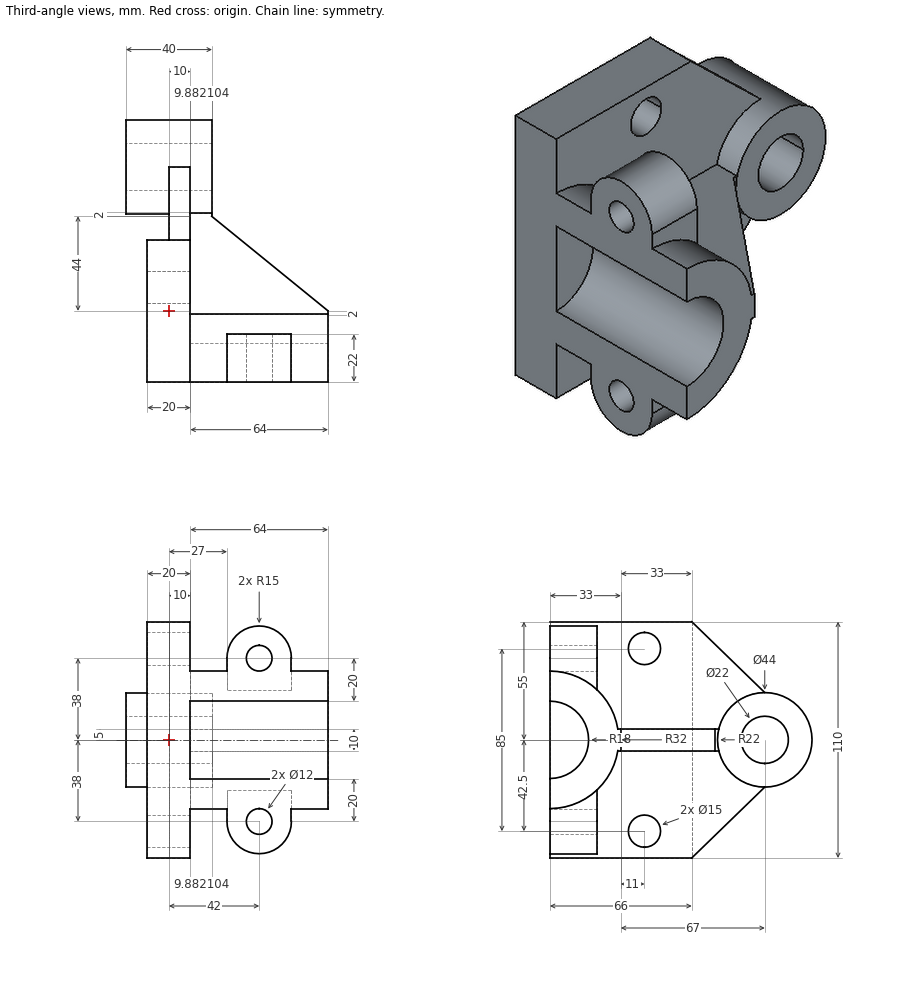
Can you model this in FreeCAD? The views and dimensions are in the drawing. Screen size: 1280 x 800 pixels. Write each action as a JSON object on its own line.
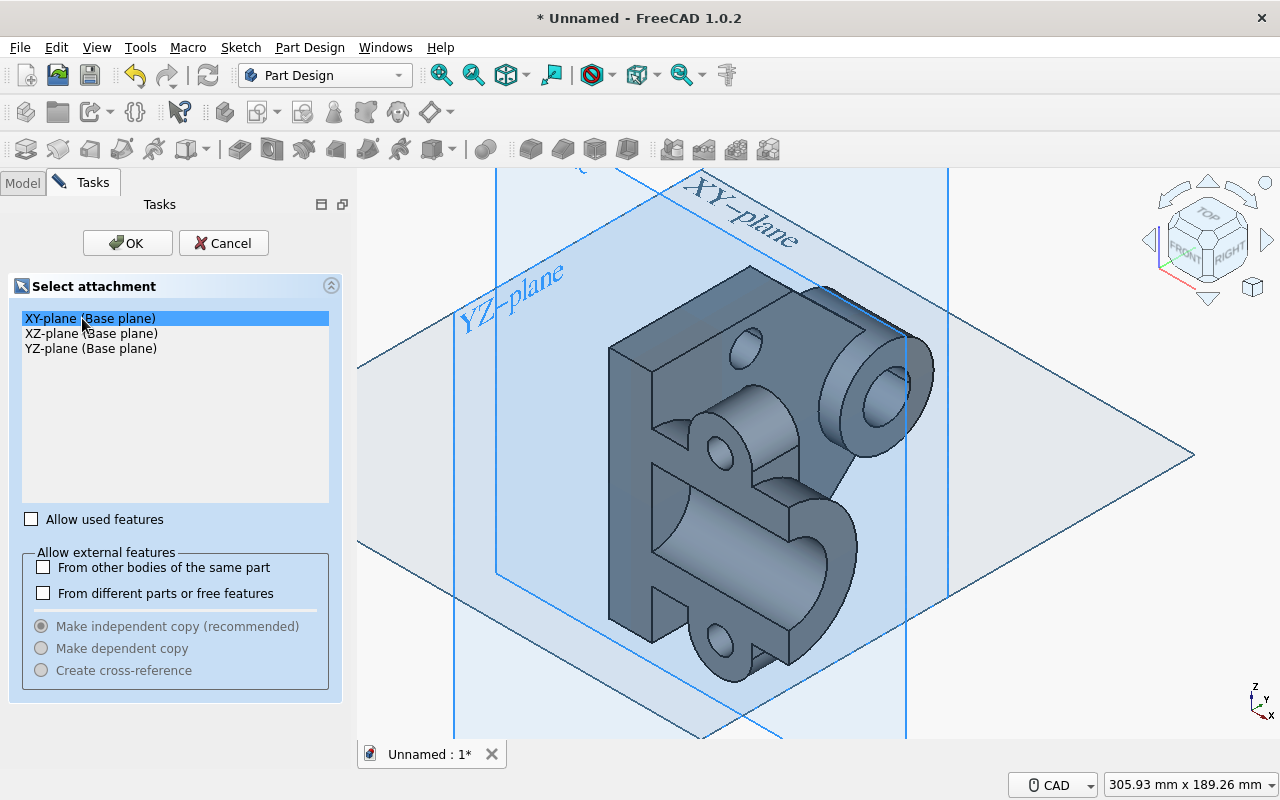
{"action": "left_click", "coordinate": [128, 243]}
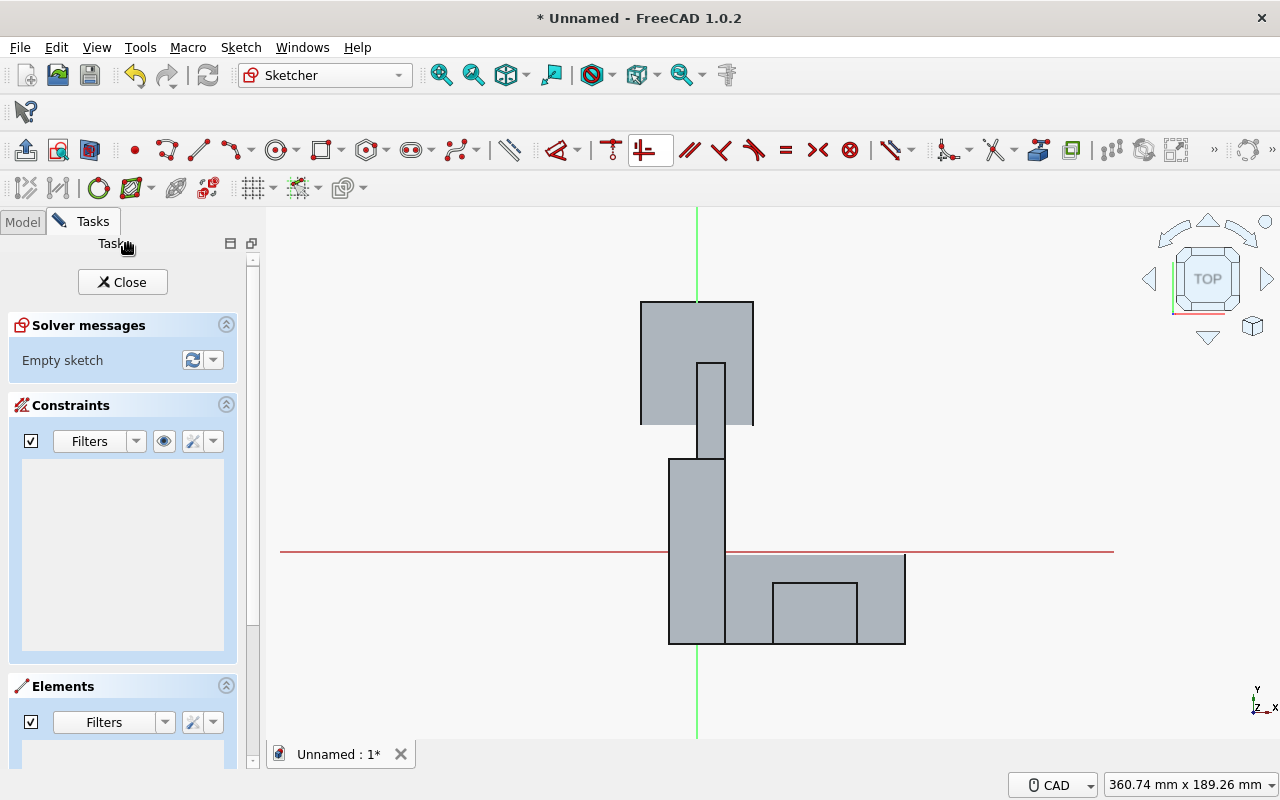
{"action": "left_click", "coordinate": [90, 150]}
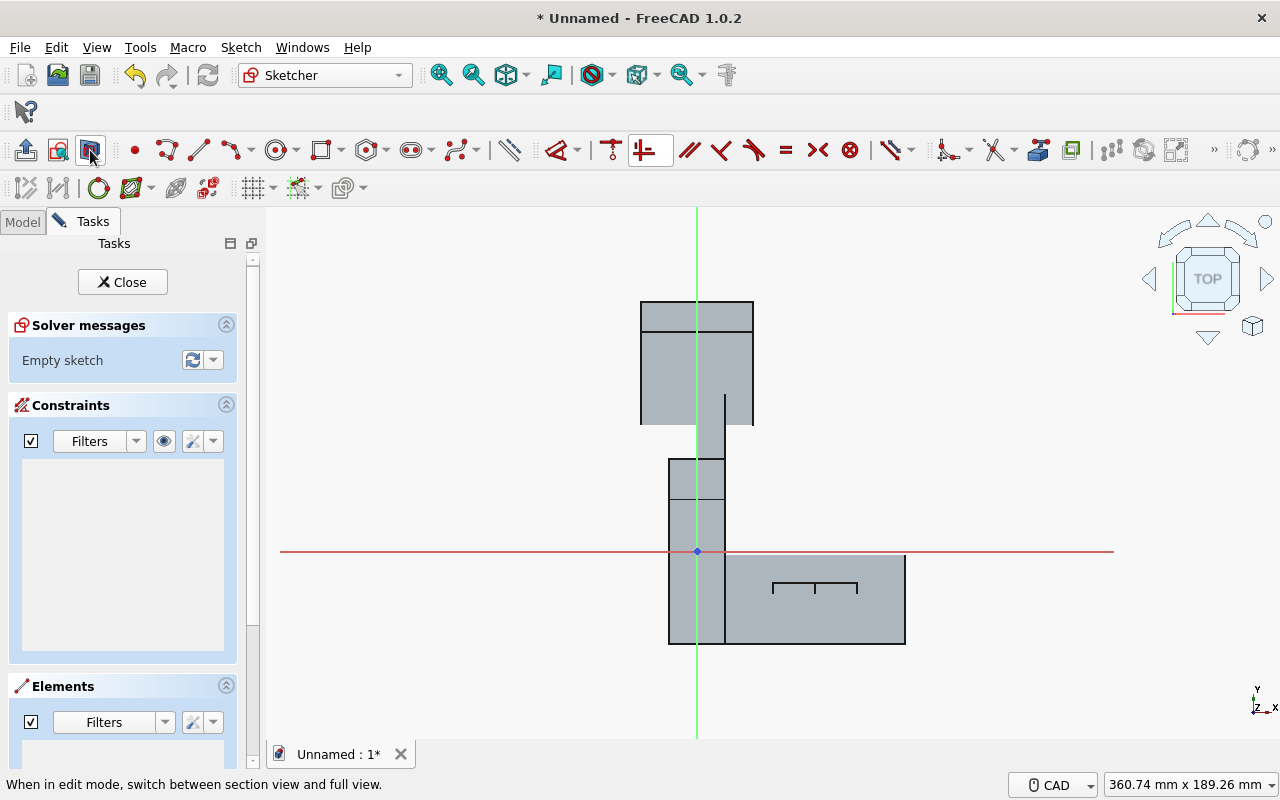
{"action": "scroll", "coordinate": [857, 500], "scroll_direction": "up", "scroll_amount": 5}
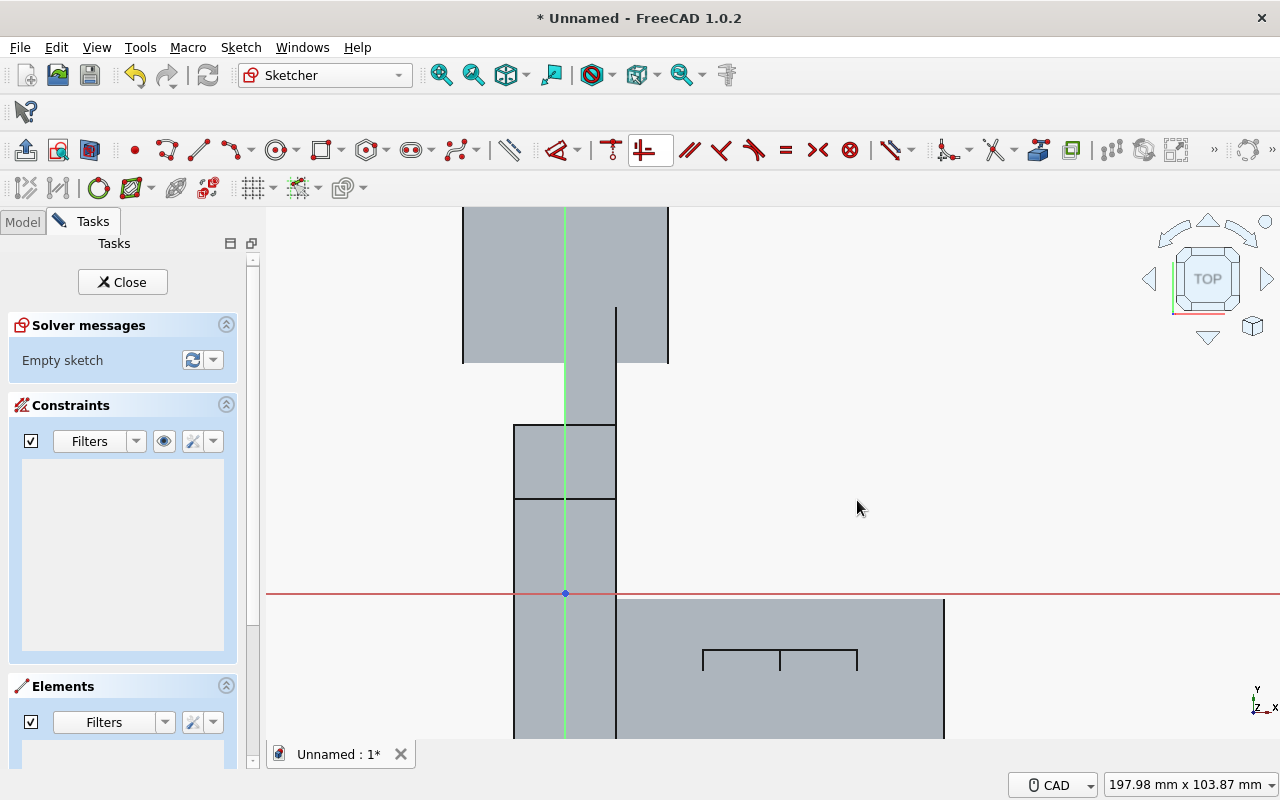
{"action": "left_click", "coordinate": [168, 150]}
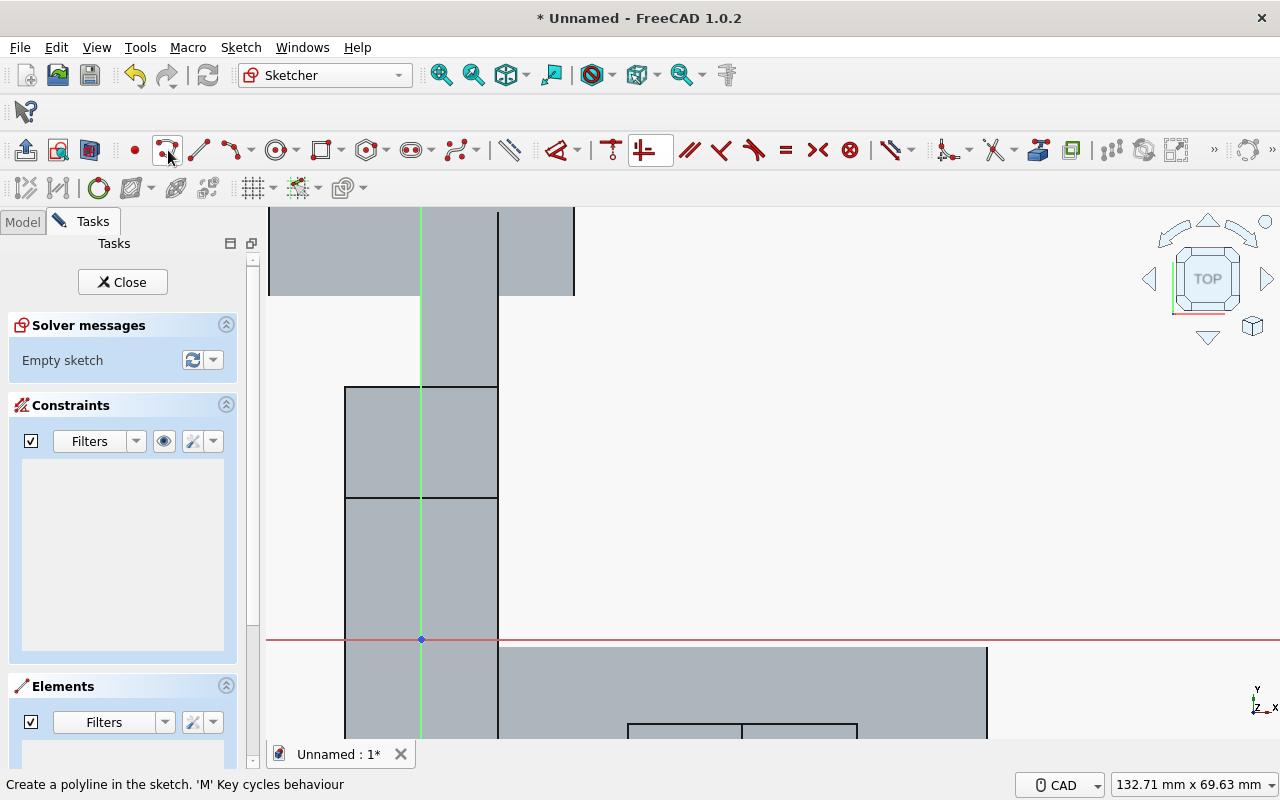
{"action": "left_click", "coordinate": [498, 640]}
{"action": "left_click", "coordinate": [987, 631]}
{"action": "left_click", "coordinate": [573, 303]}
{"action": "left_click", "coordinate": [498, 303]}
{"action": "left_click", "coordinate": [498, 640]}
{"action": "key", "text": "Escape"}
{"action": "key", "text": "Escape"}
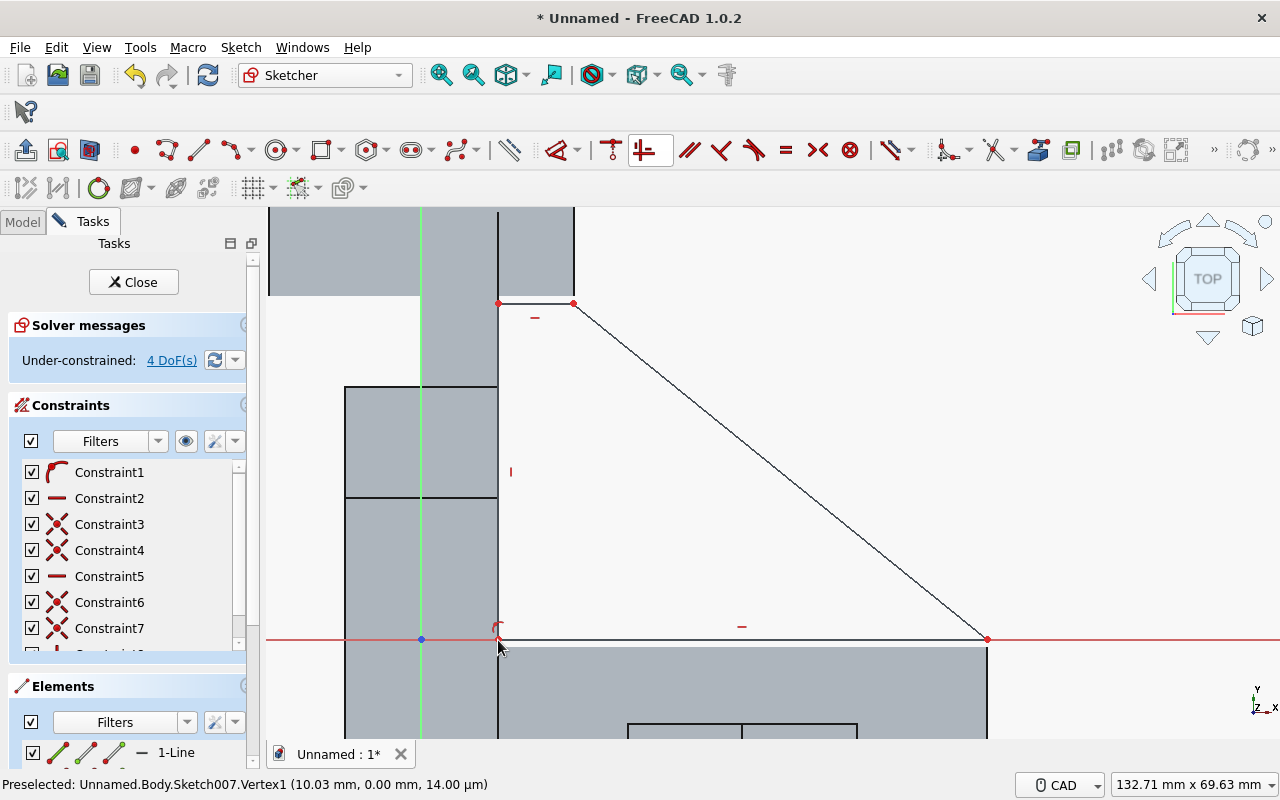
{"action": "left_click", "coordinate": [556, 150]}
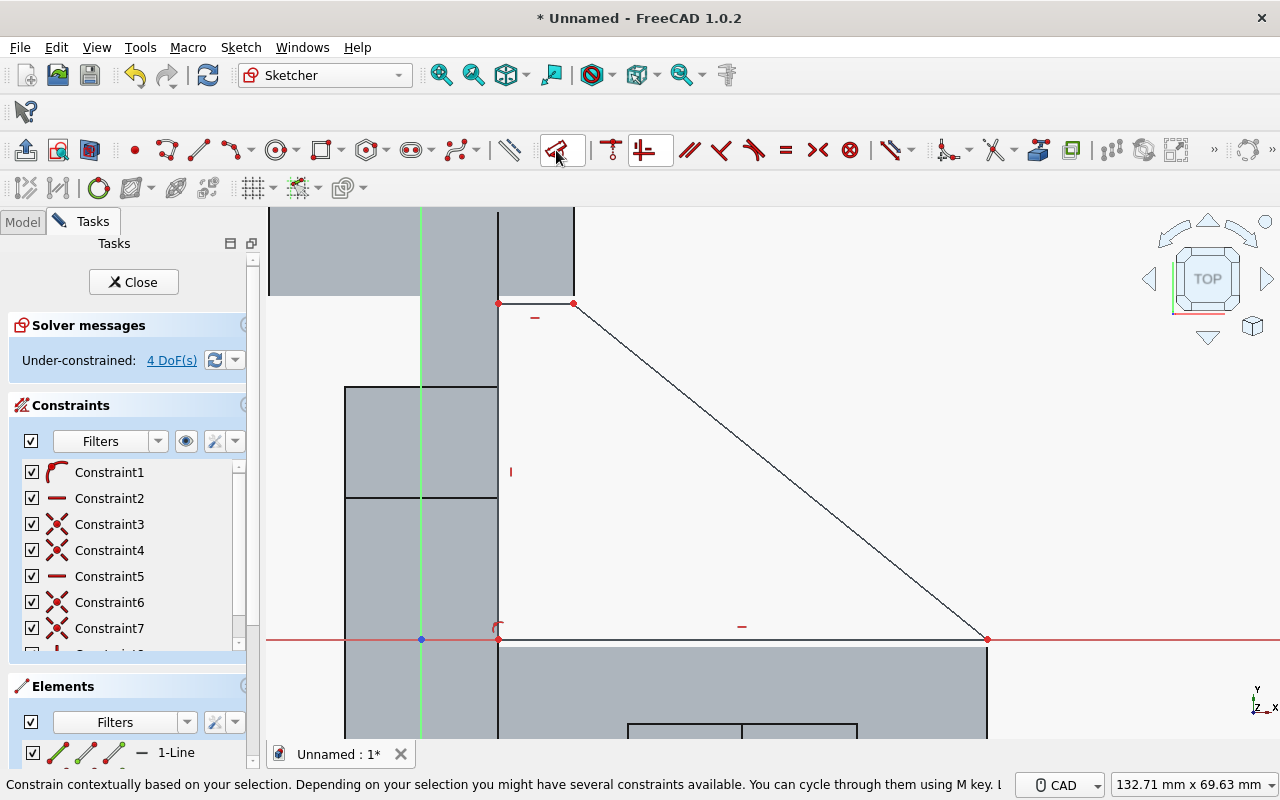
{"action": "left_click", "coordinate": [645, 640]}
{"action": "left_click", "coordinate": [743, 674]}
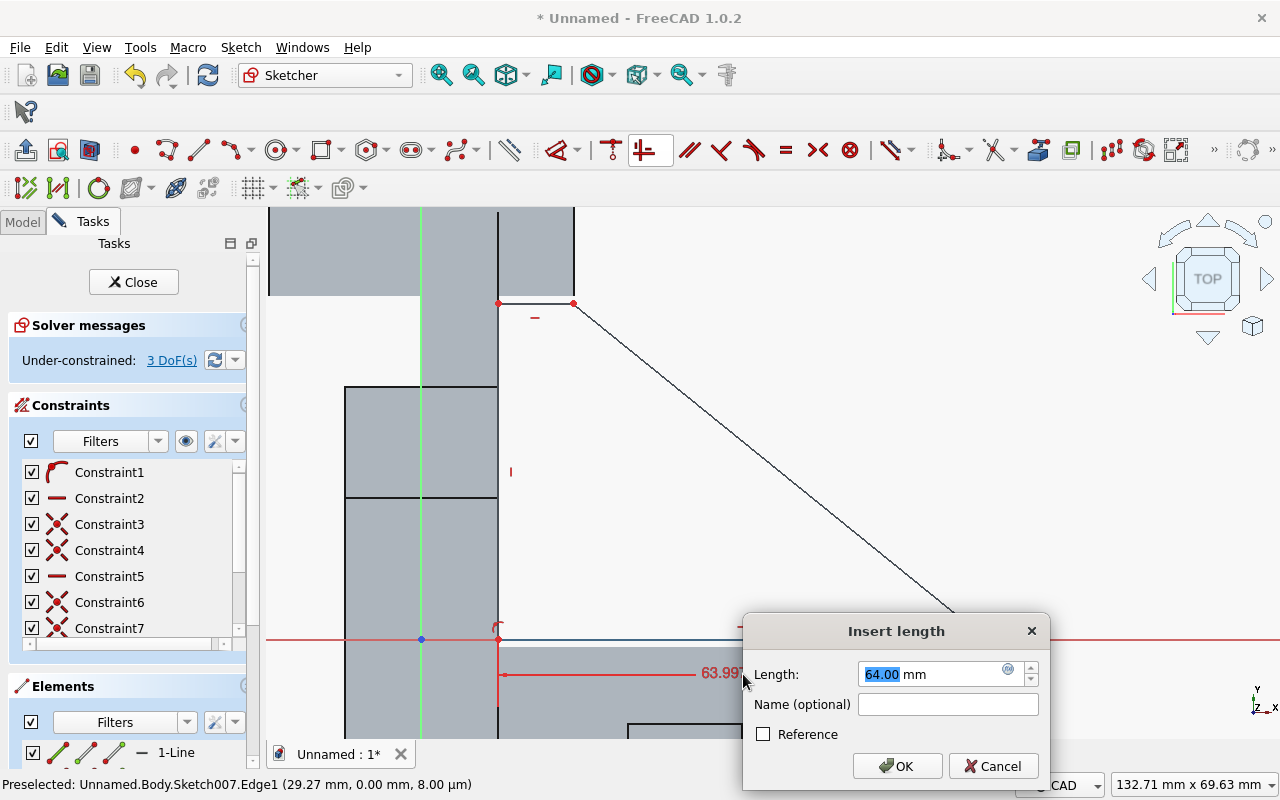
{"action": "type", "text": "64"}
{"action": "key", "text": "Return"}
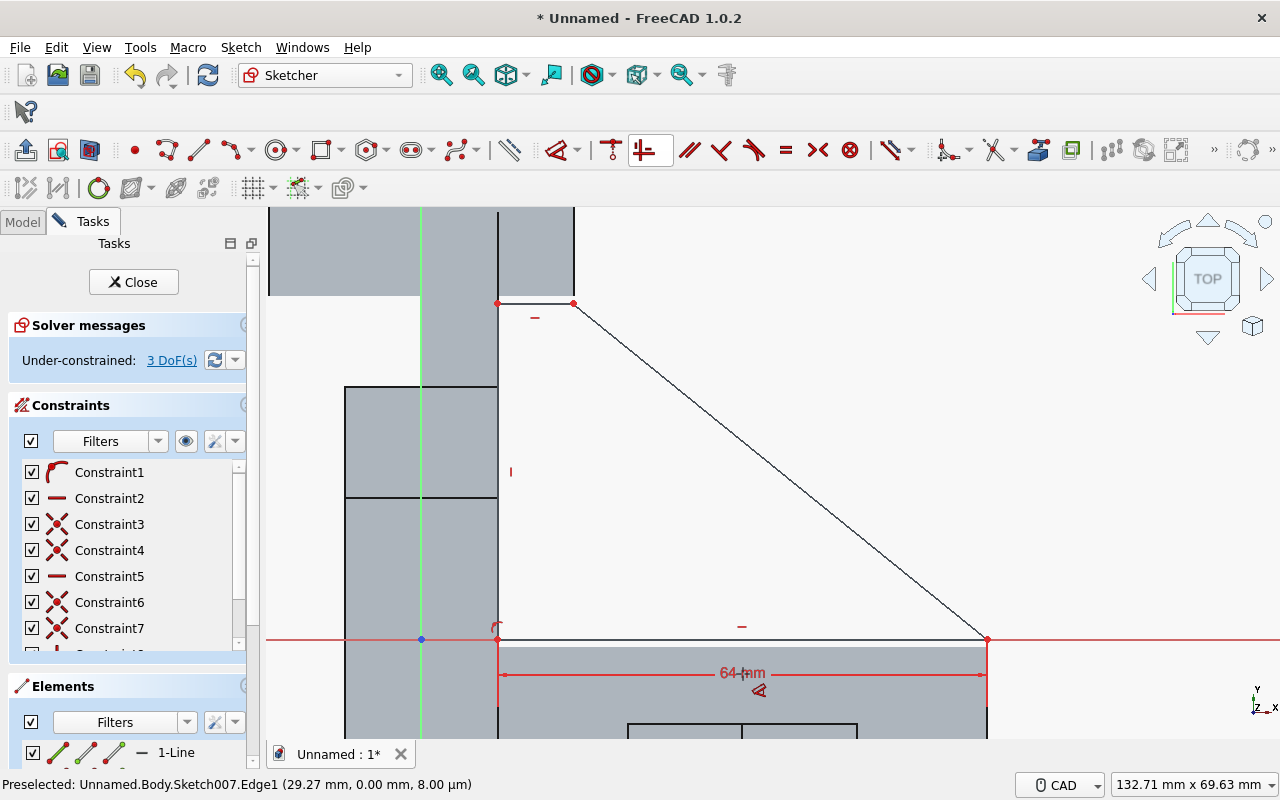
{"action": "left_click", "coordinate": [498, 405]}
{"action": "left_click", "coordinate": [464, 472]}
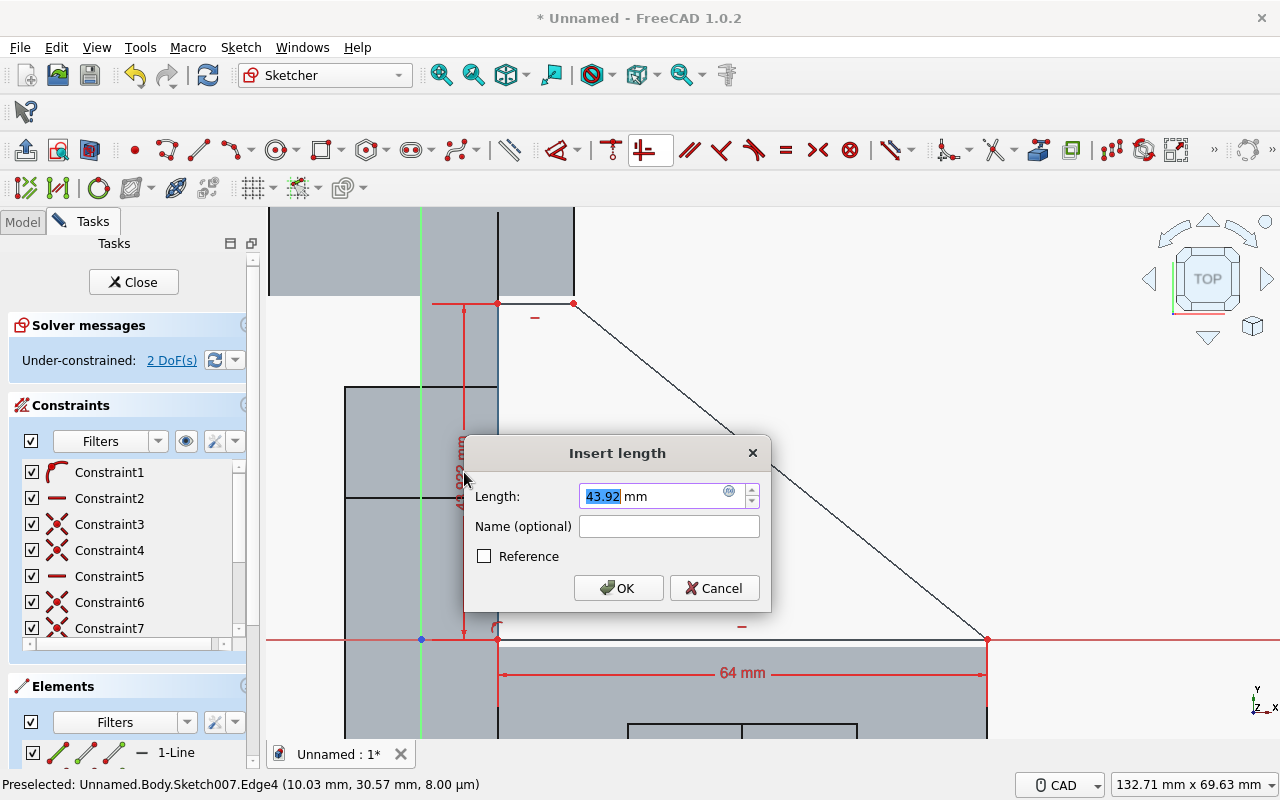
{"action": "type", "text": "44"}
{"action": "key", "text": "Return"}